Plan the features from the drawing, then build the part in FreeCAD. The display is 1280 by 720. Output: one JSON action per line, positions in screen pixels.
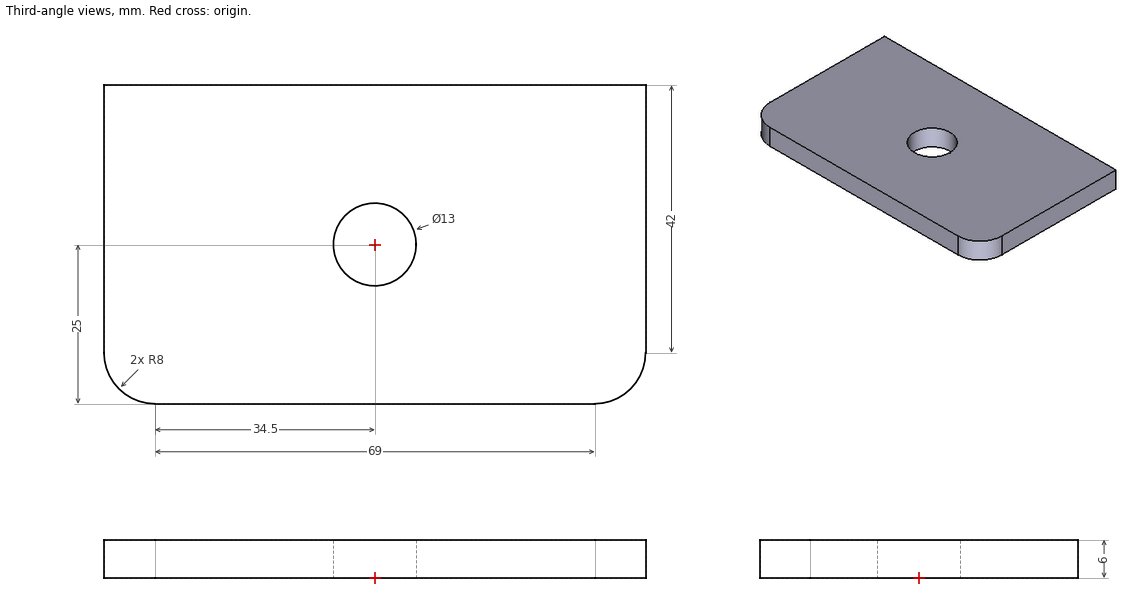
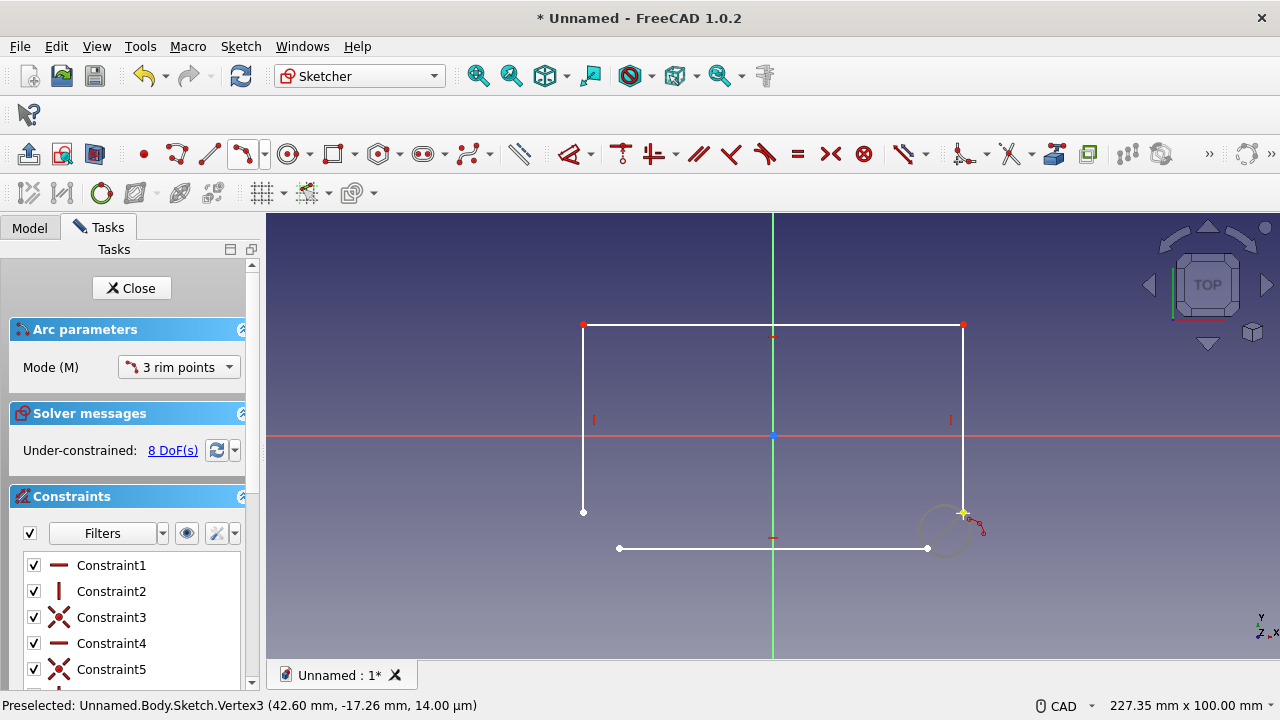
{"action": "scroll", "coordinate": [952, 537], "scroll_direction": "up", "scroll_amount": 3}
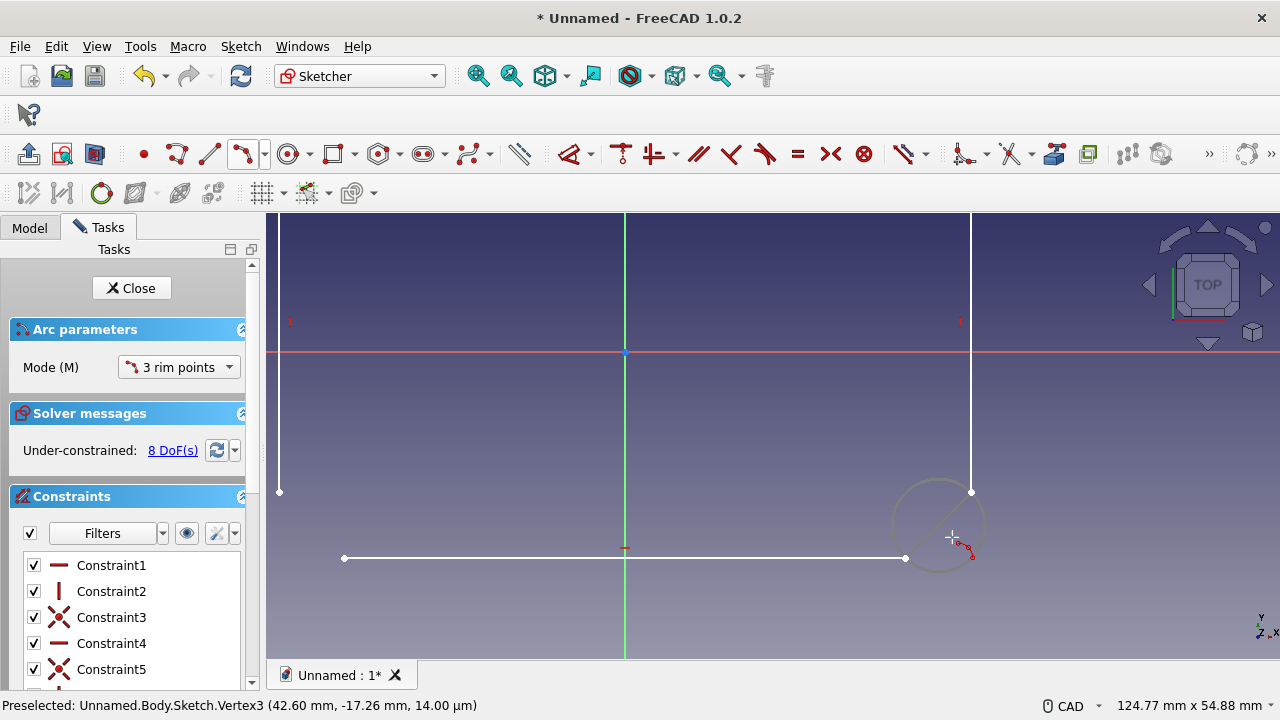
{"action": "left_click", "coordinate": [952, 536]}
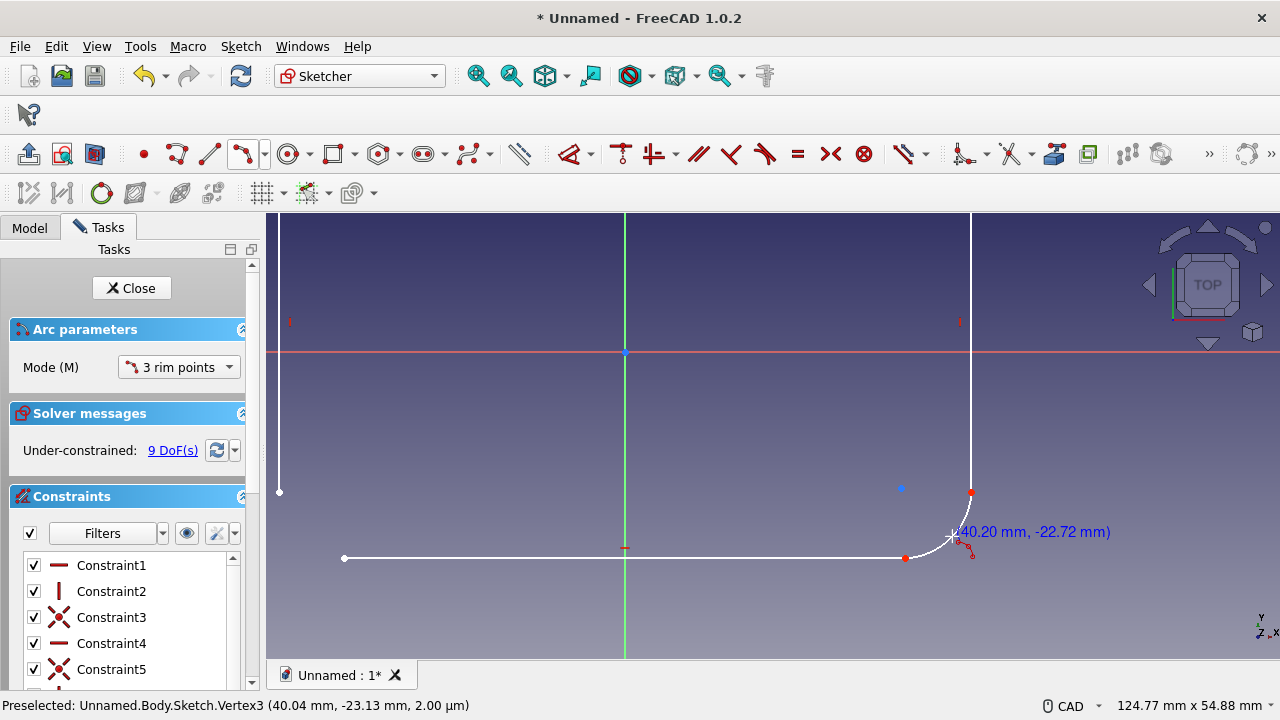
{"action": "scroll", "coordinate": [866, 606], "scroll_direction": "down", "scroll_amount": 2}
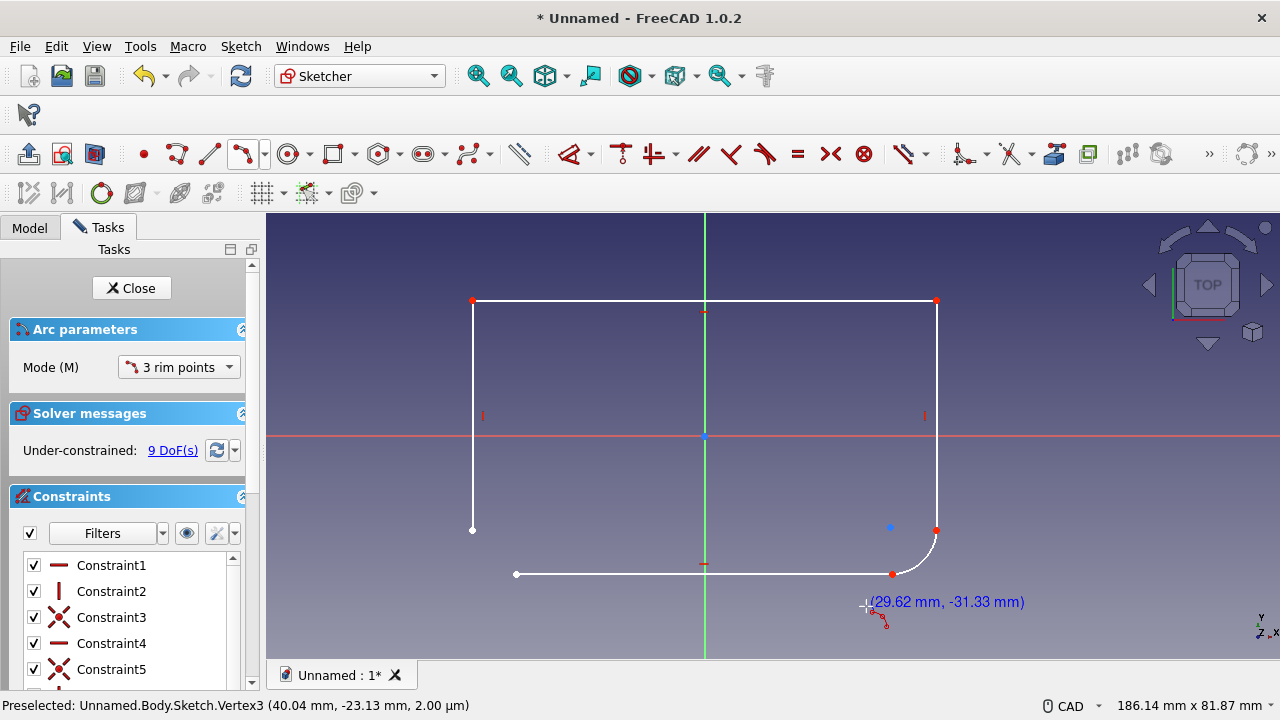
{"action": "left_click", "coordinate": [473, 530]}
{"action": "left_click", "coordinate": [517, 574]}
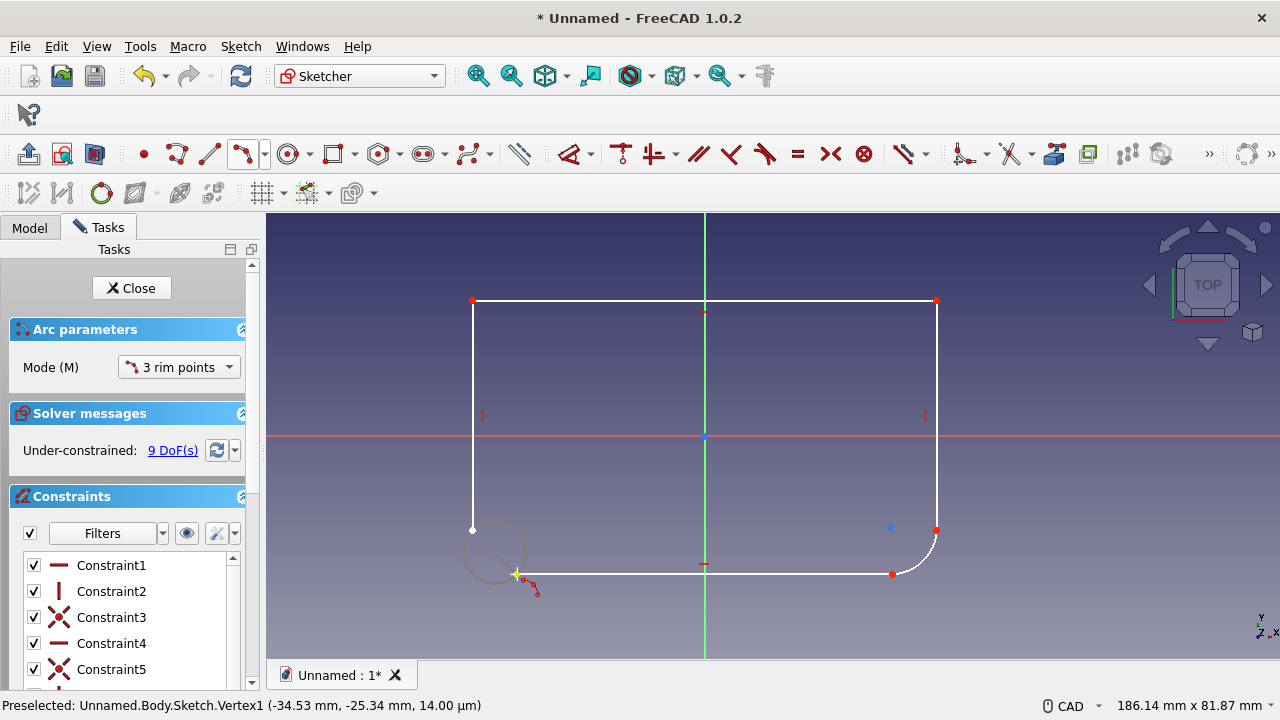
{"action": "scroll", "coordinate": [486, 560], "scroll_direction": "up", "scroll_amount": 2}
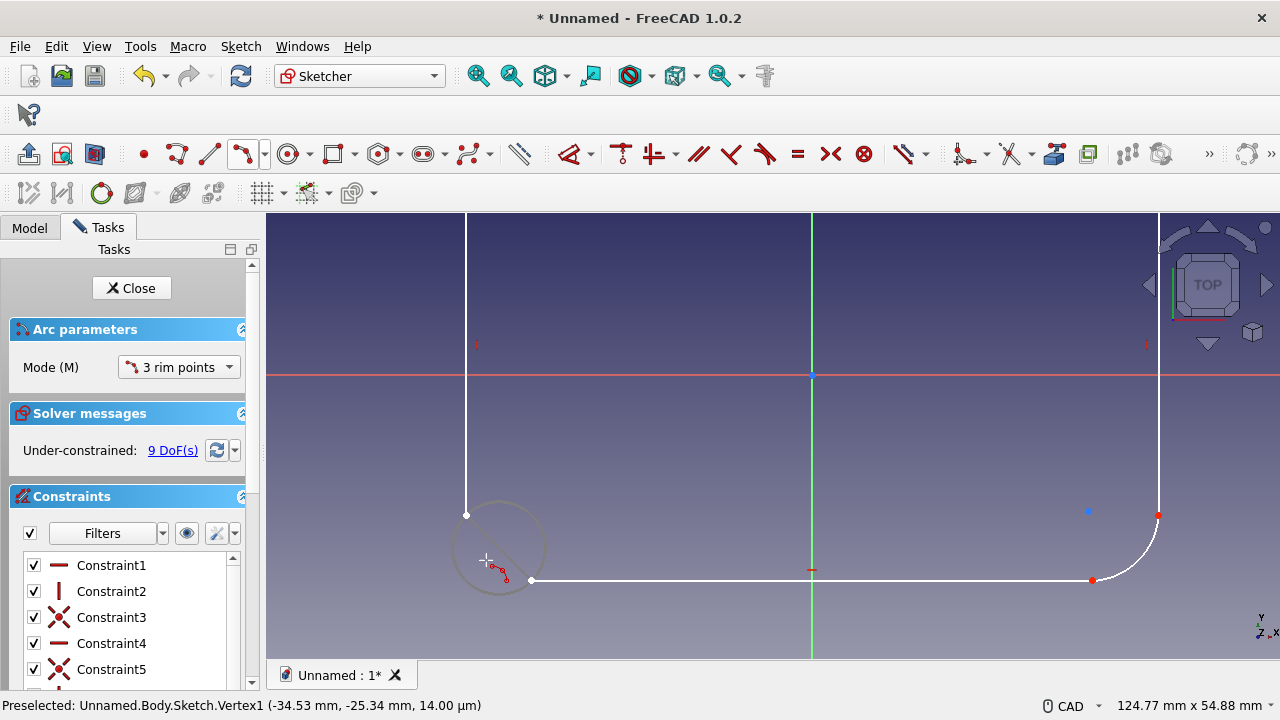
{"action": "left_click", "coordinate": [486, 559]}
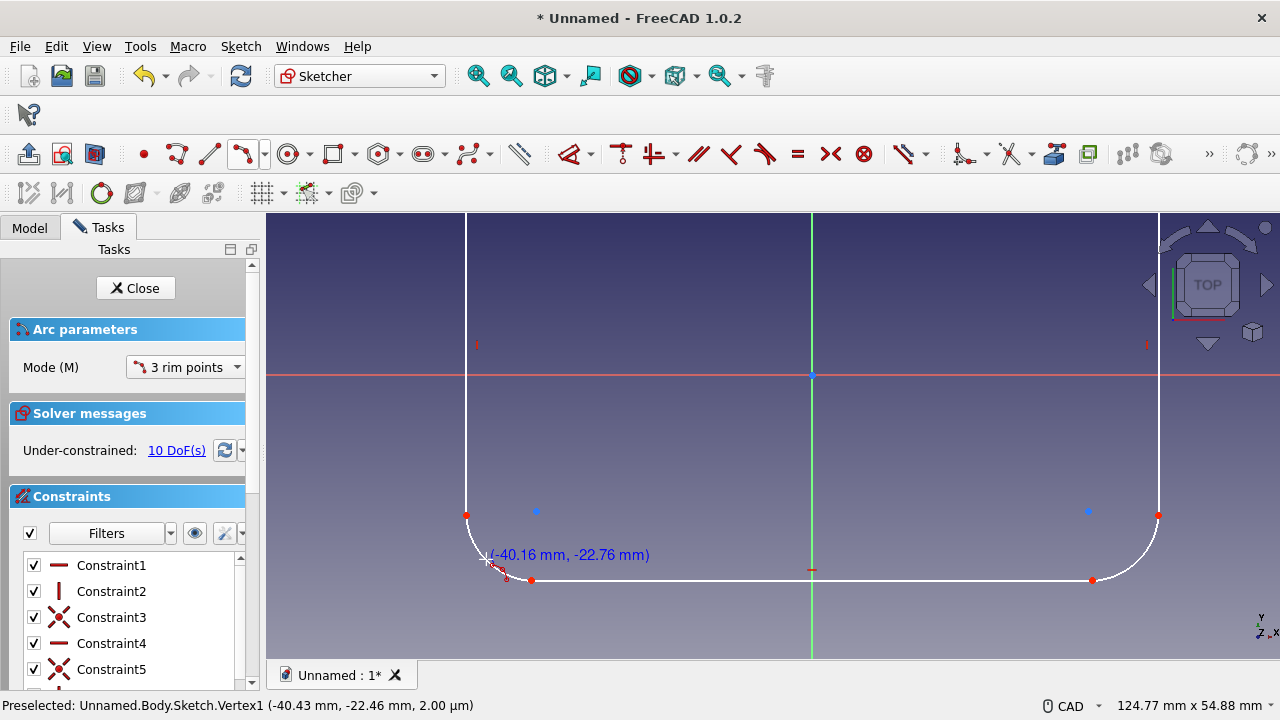
{"action": "left_click", "coordinate": [288, 154]}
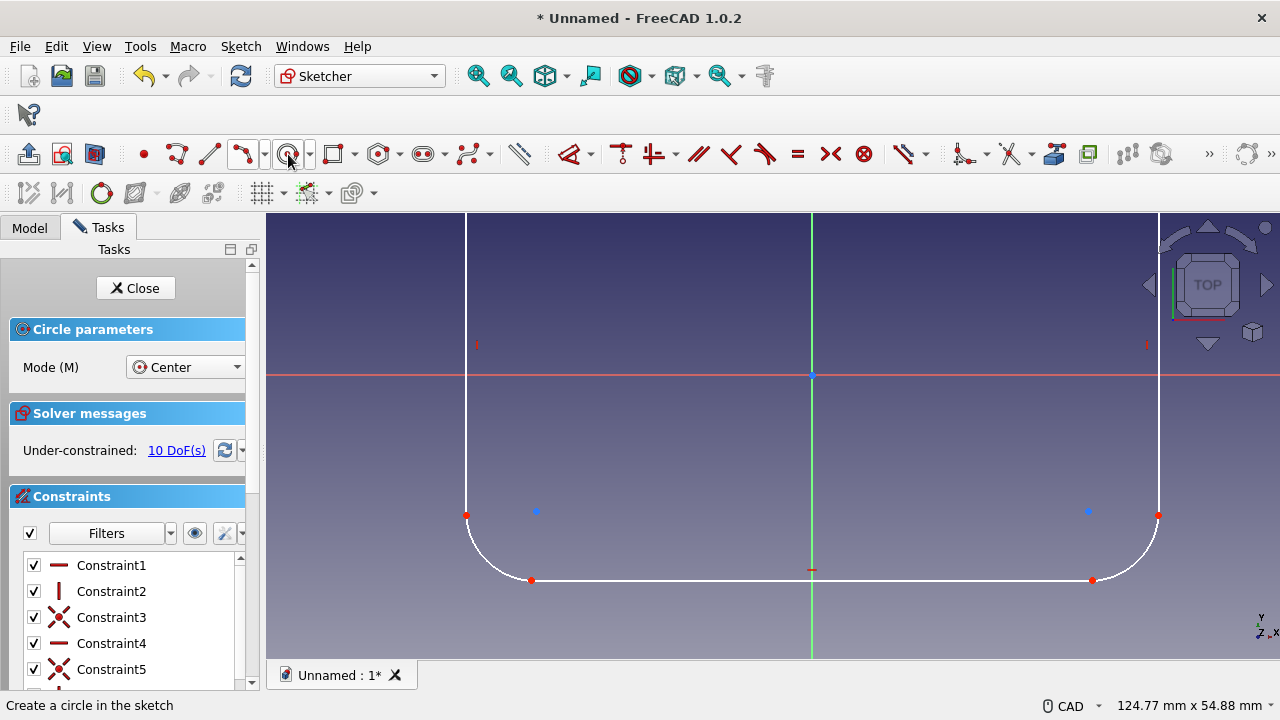
{"action": "left_click", "coordinate": [812, 375]}
{"action": "mouse_move", "coordinate": [850, 338]}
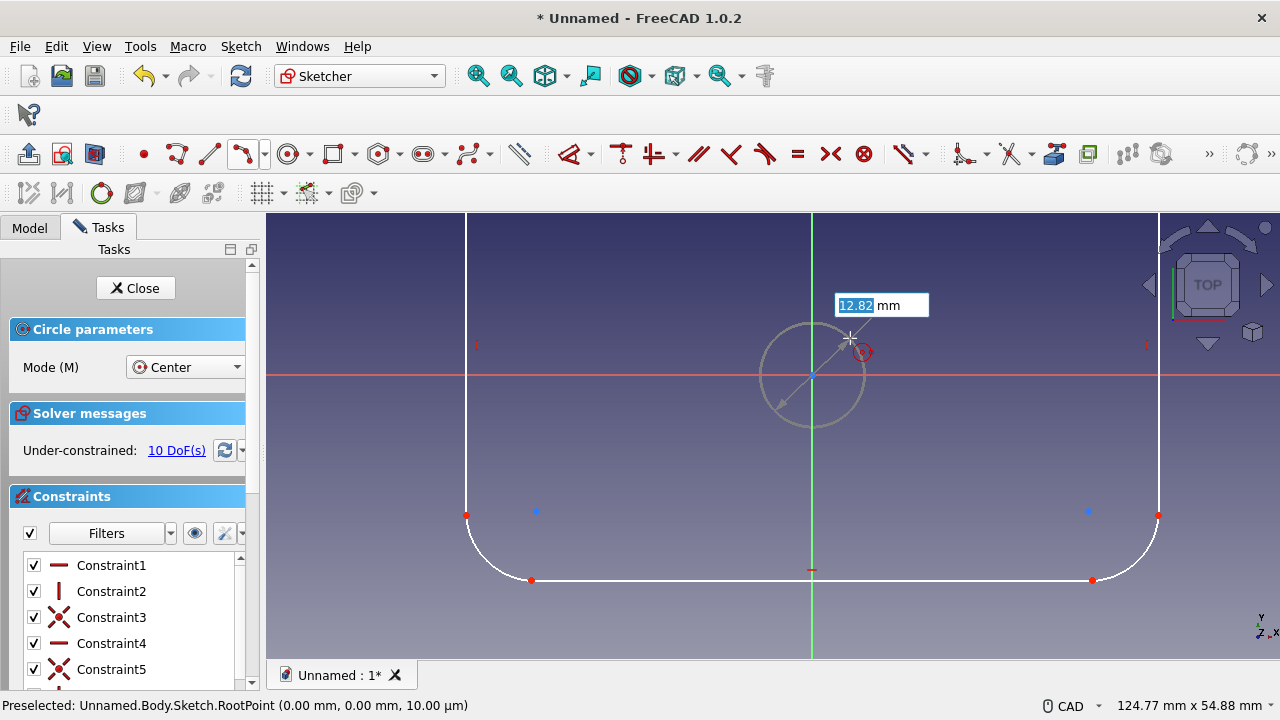
{"action": "type", "text": "13"}
{"action": "key", "text": "Return"}
{"action": "key", "text": "Escape"}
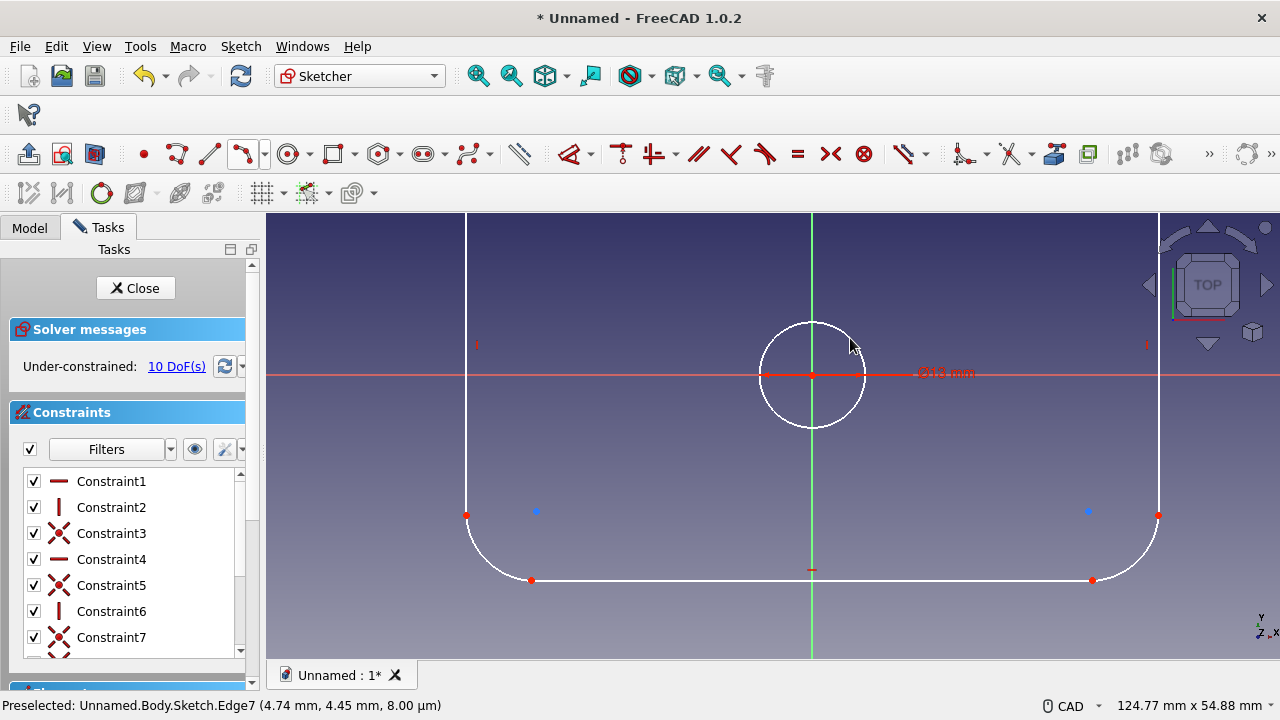
{"action": "left_click", "coordinate": [700, 581]}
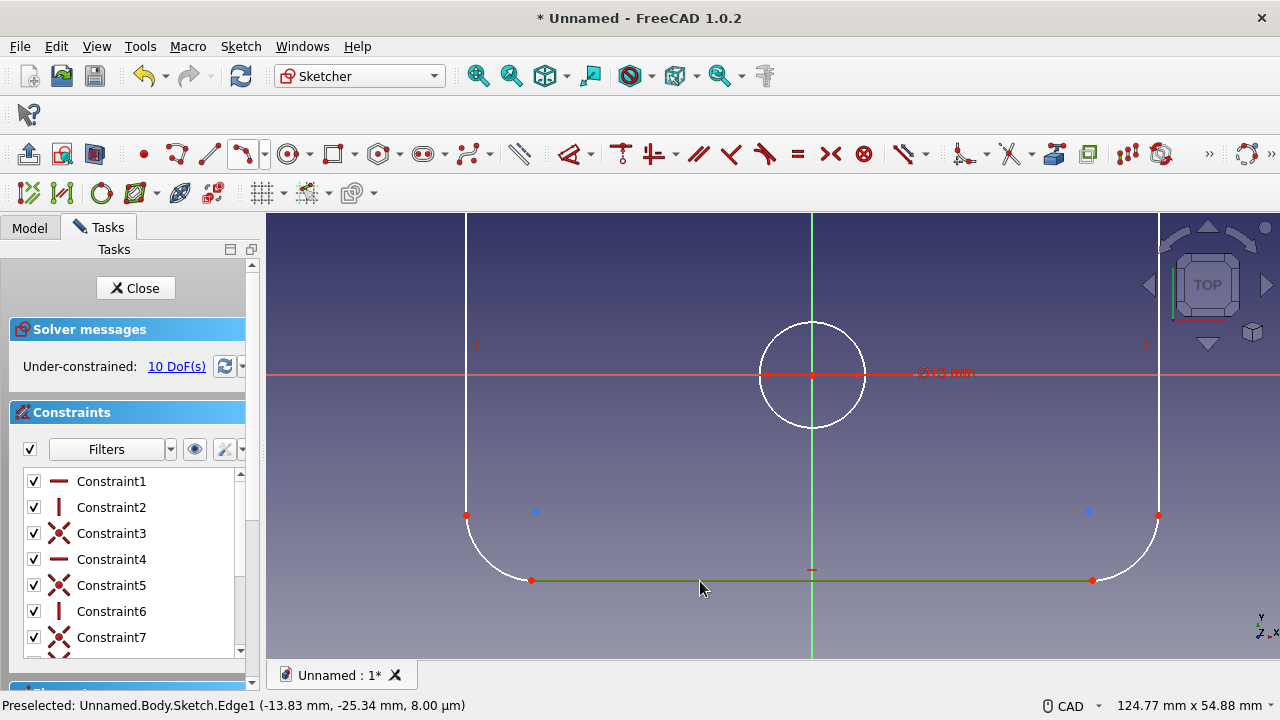
{"action": "left_click", "coordinate": [1113, 577]}